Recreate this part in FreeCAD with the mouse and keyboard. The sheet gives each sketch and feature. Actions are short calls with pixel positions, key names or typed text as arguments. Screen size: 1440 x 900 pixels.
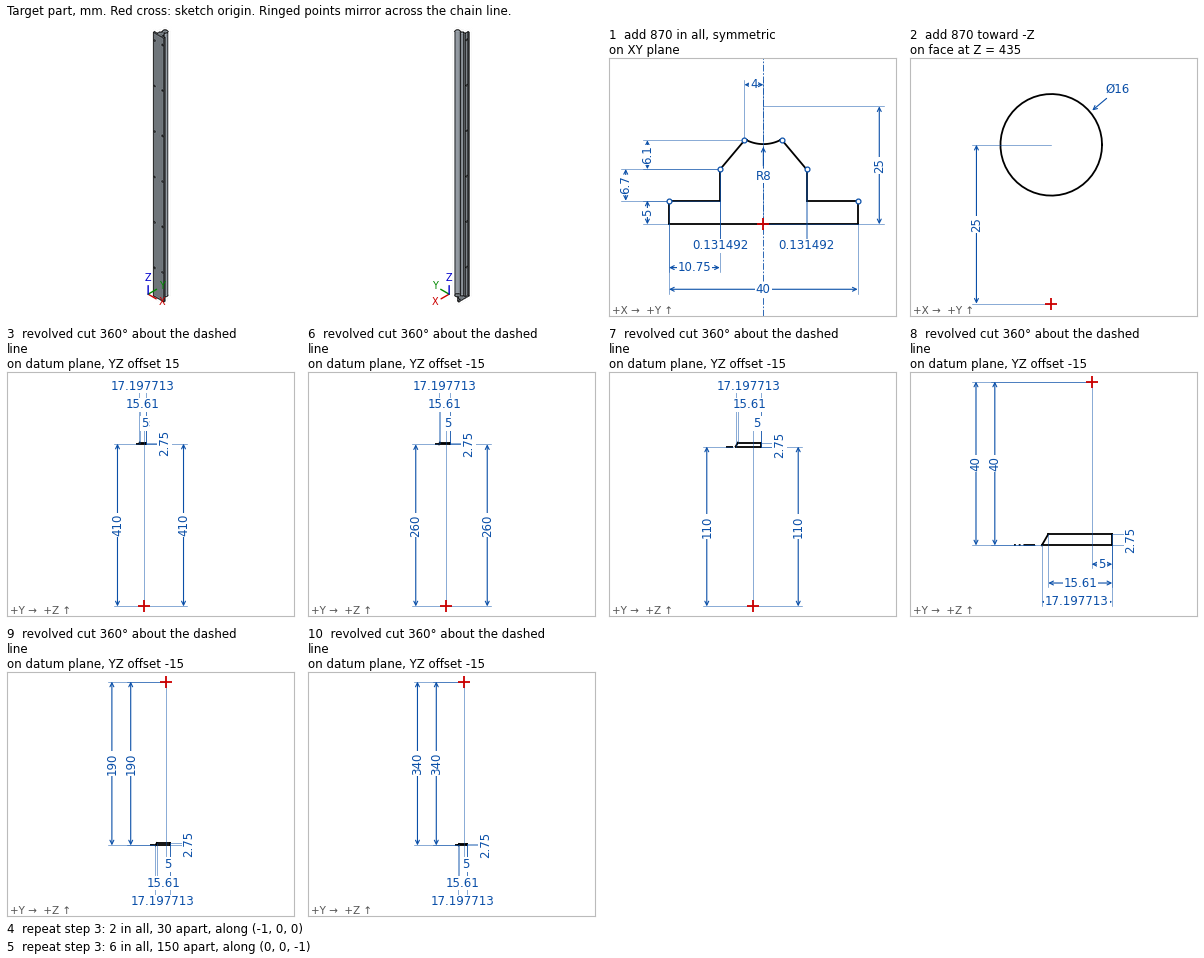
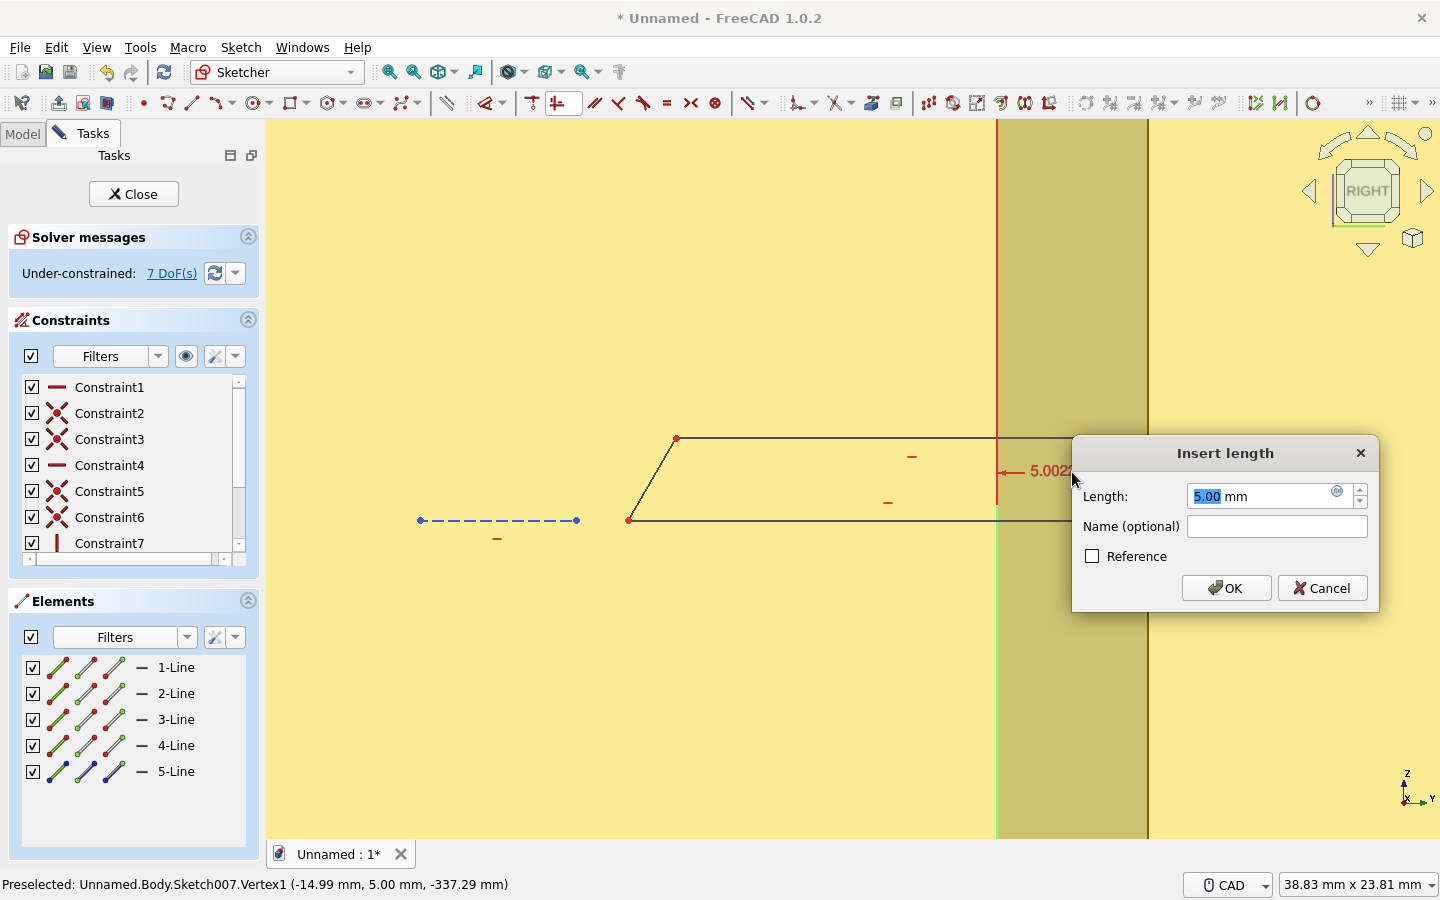
text(5)
key(Return)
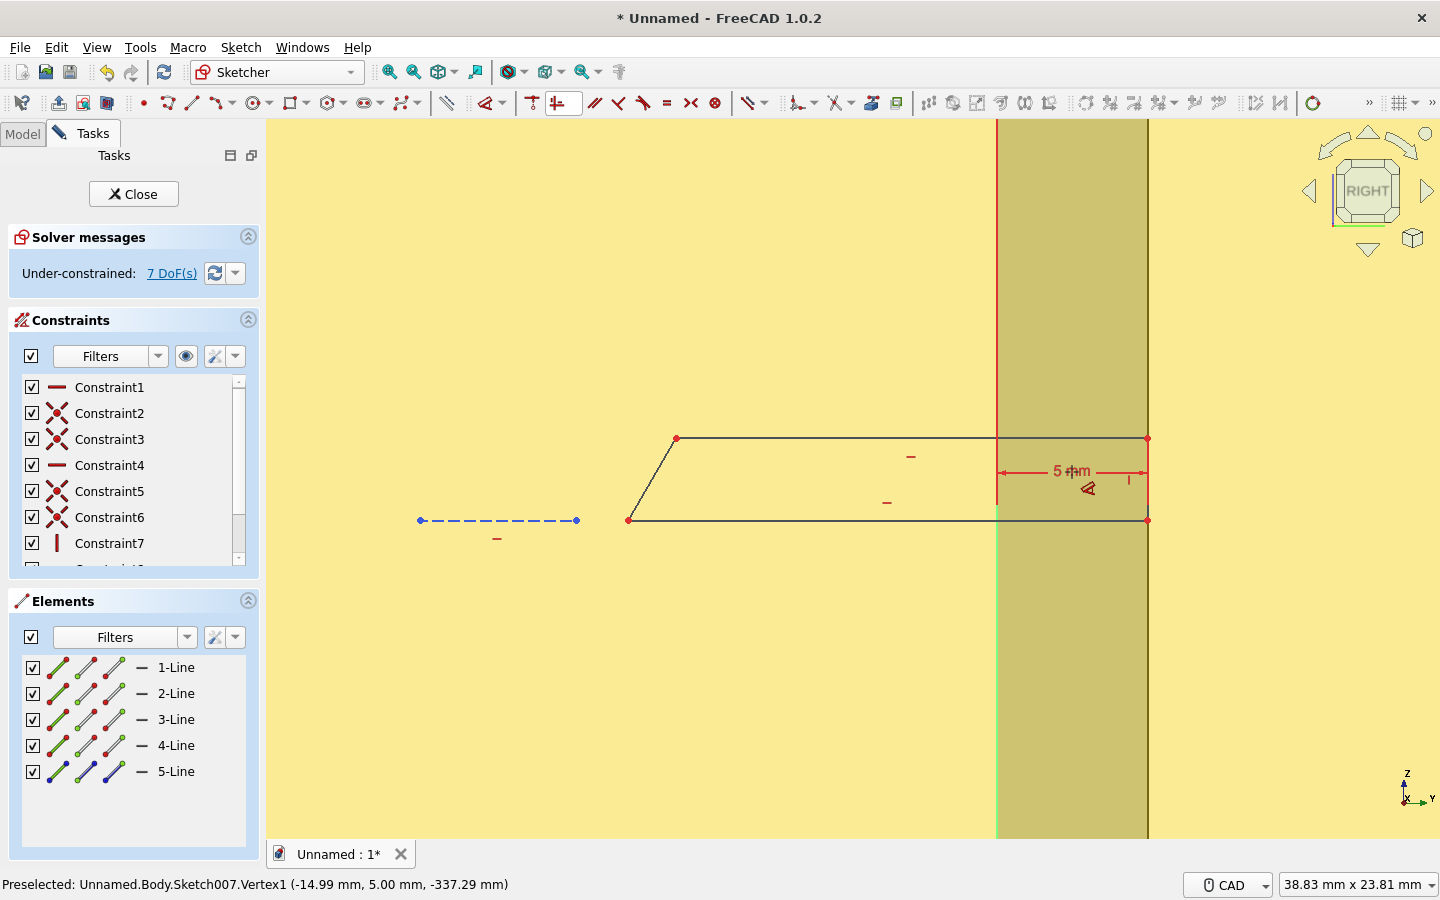
click(1148, 496)
click(1182, 480)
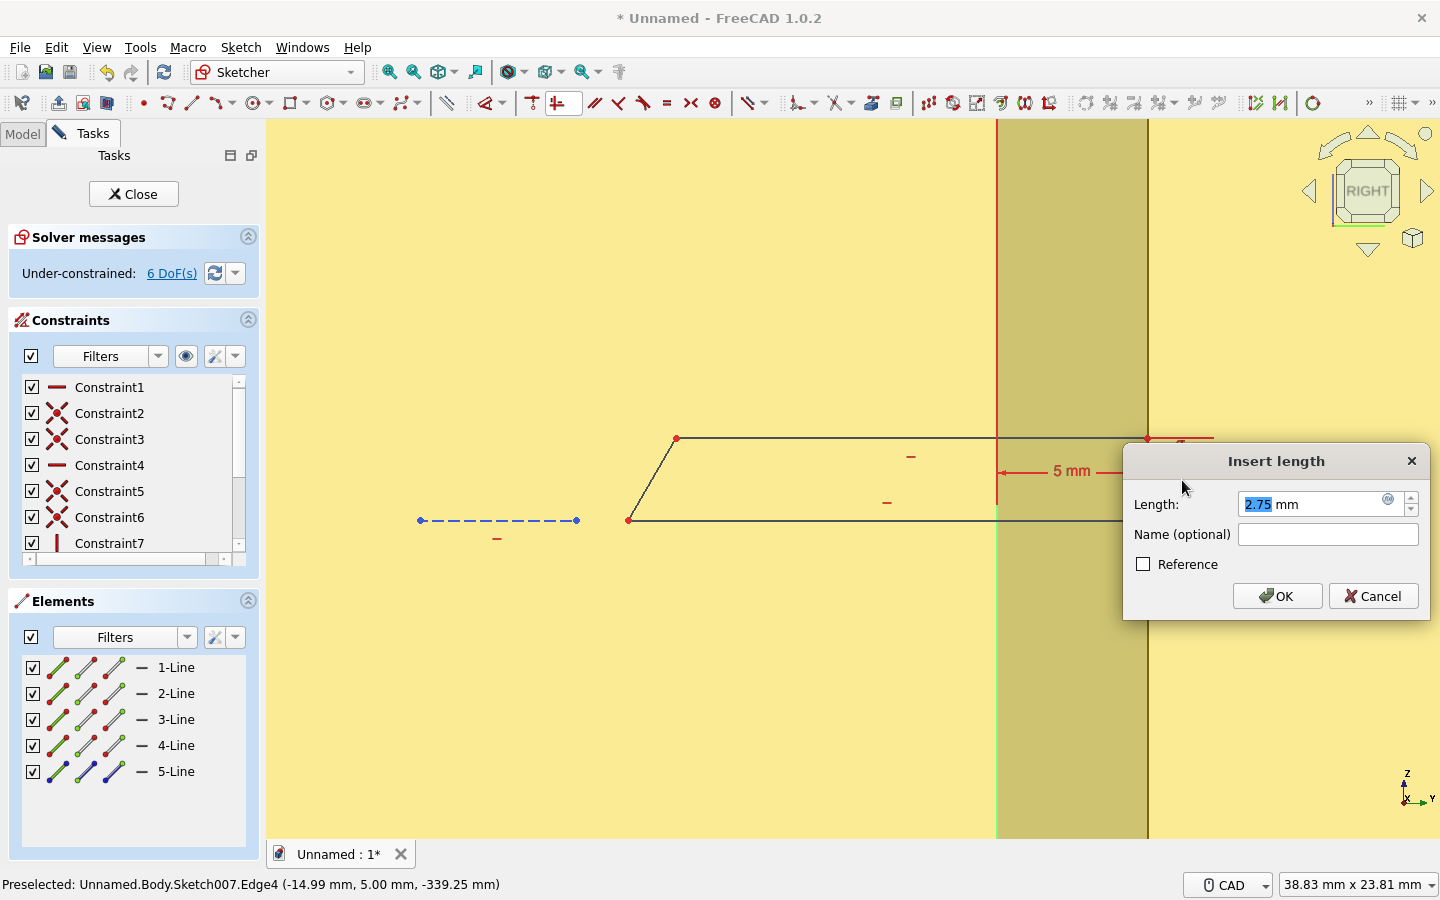
text(2.75)
key(Return)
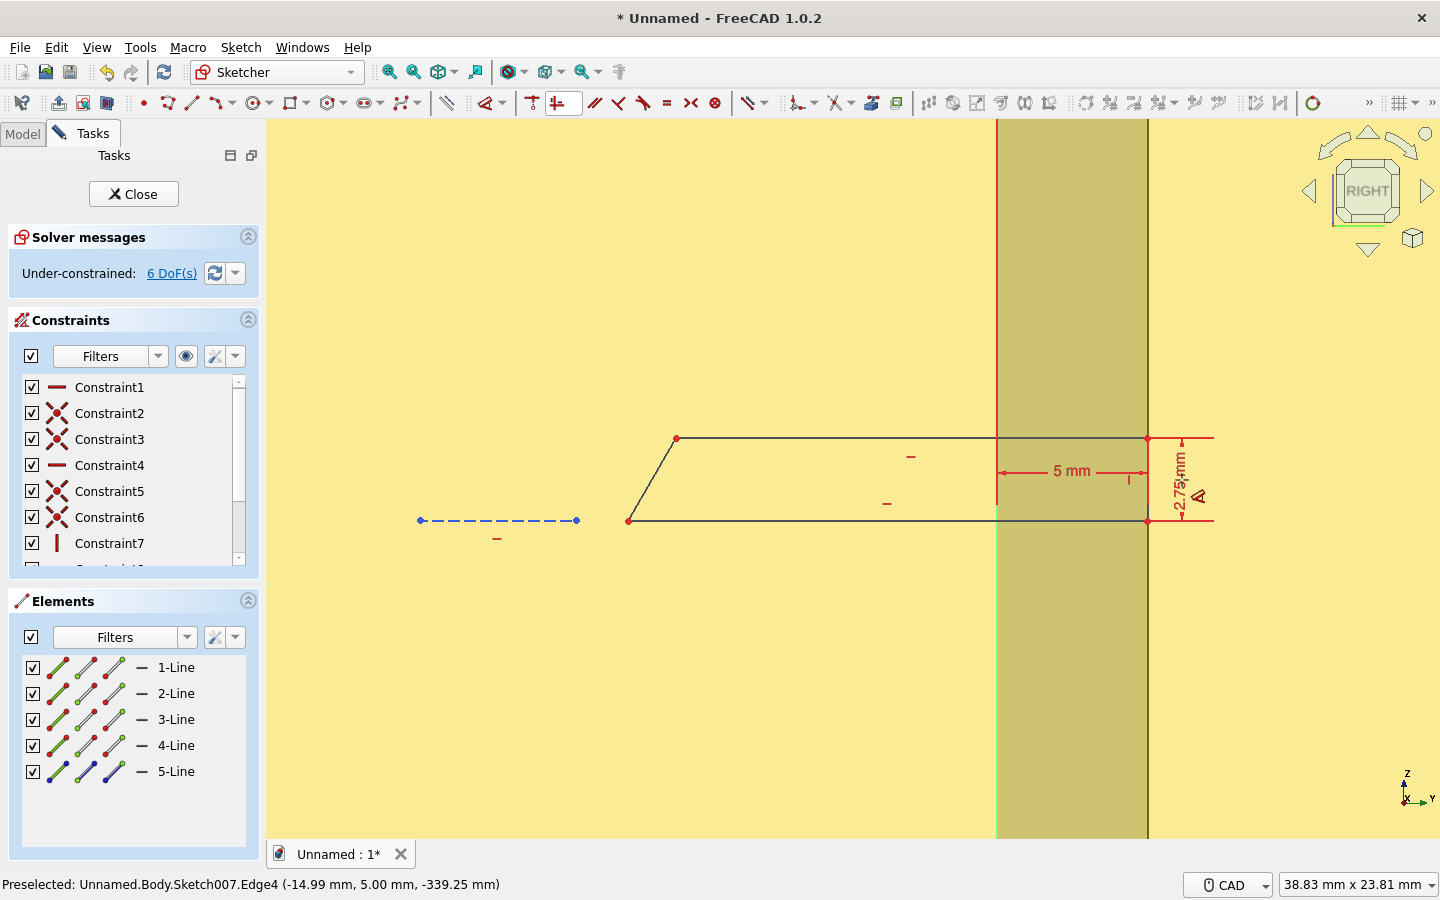
click(628, 521)
click(1031, 334)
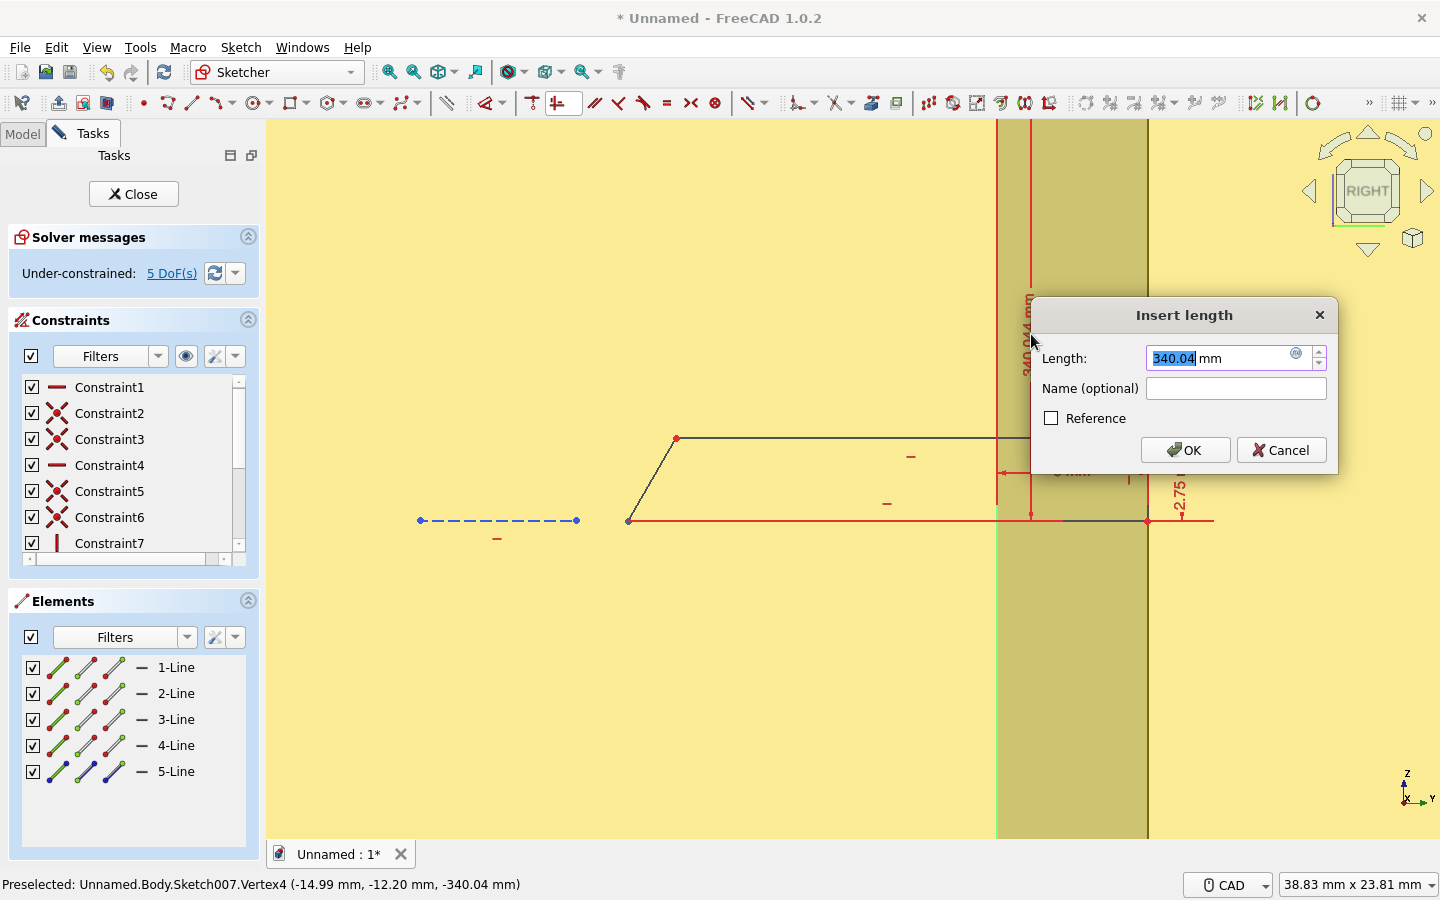
text(340)
key(Return)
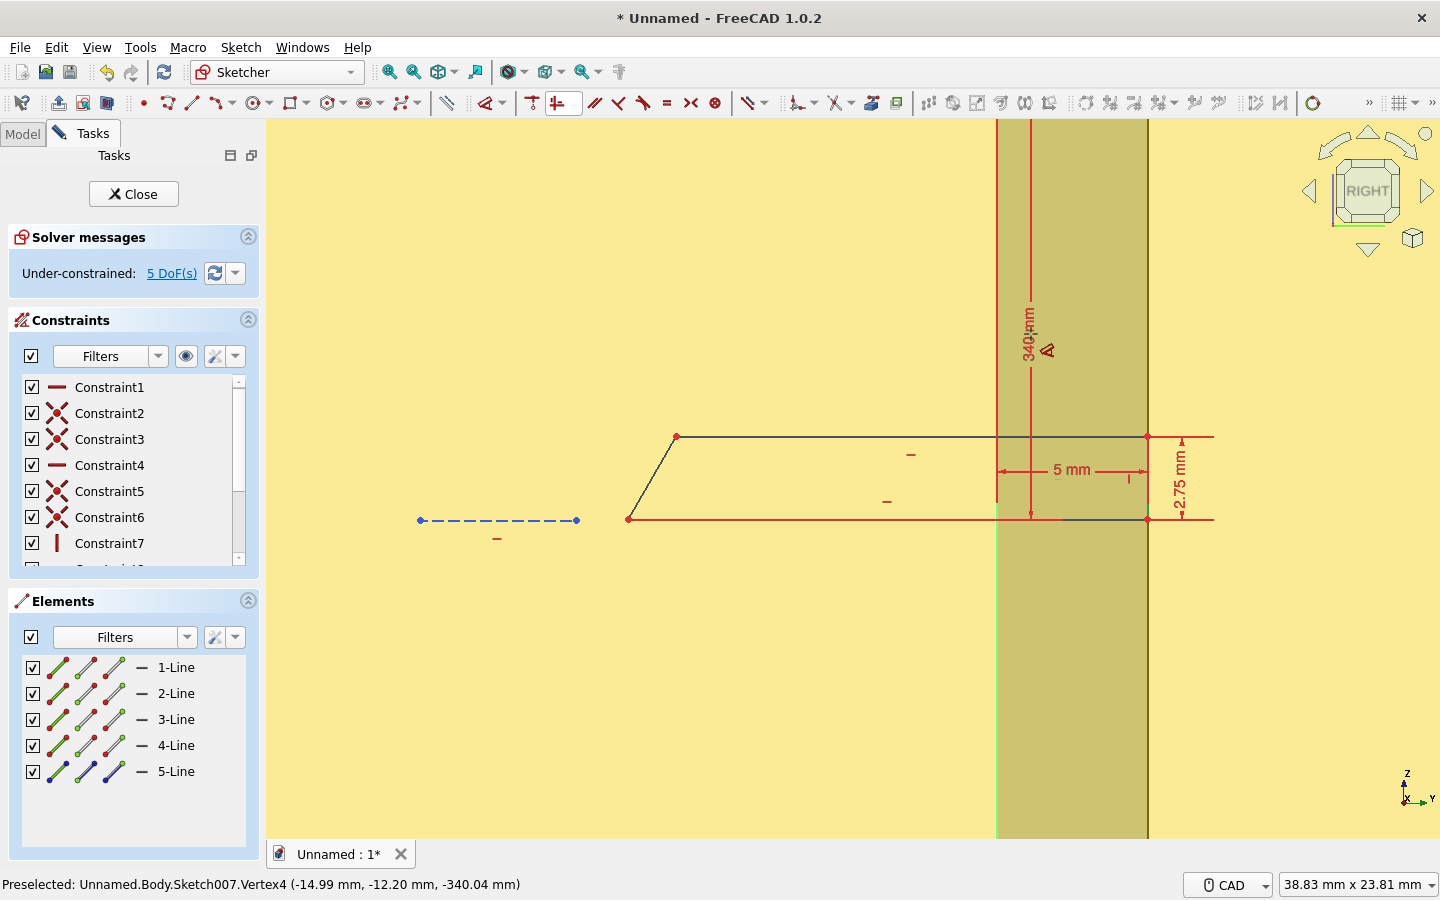
click(576, 521)
click(1031, 248)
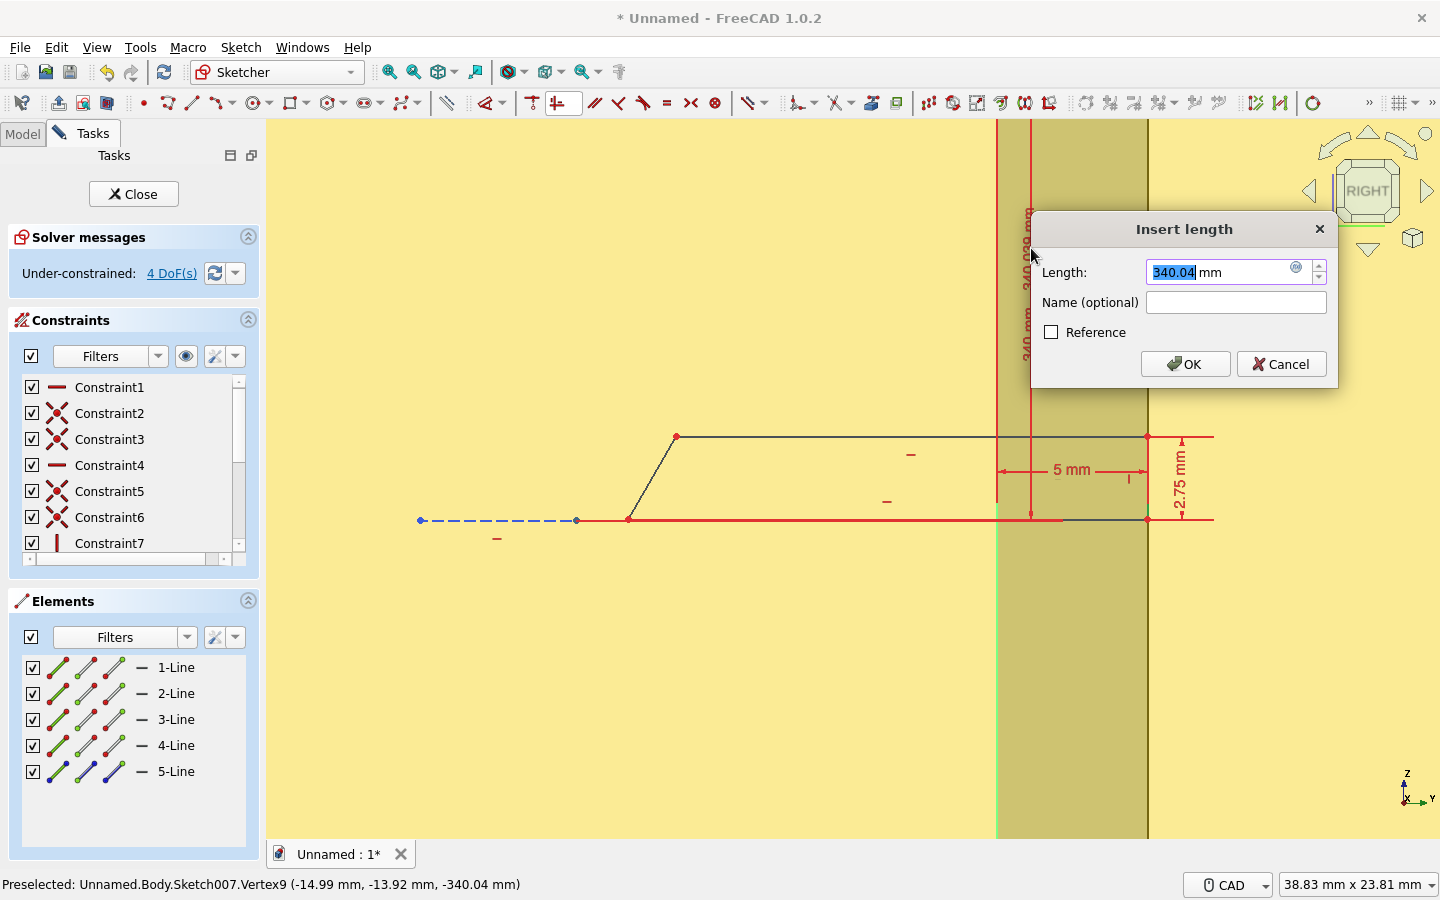
text(340)
key(Return)